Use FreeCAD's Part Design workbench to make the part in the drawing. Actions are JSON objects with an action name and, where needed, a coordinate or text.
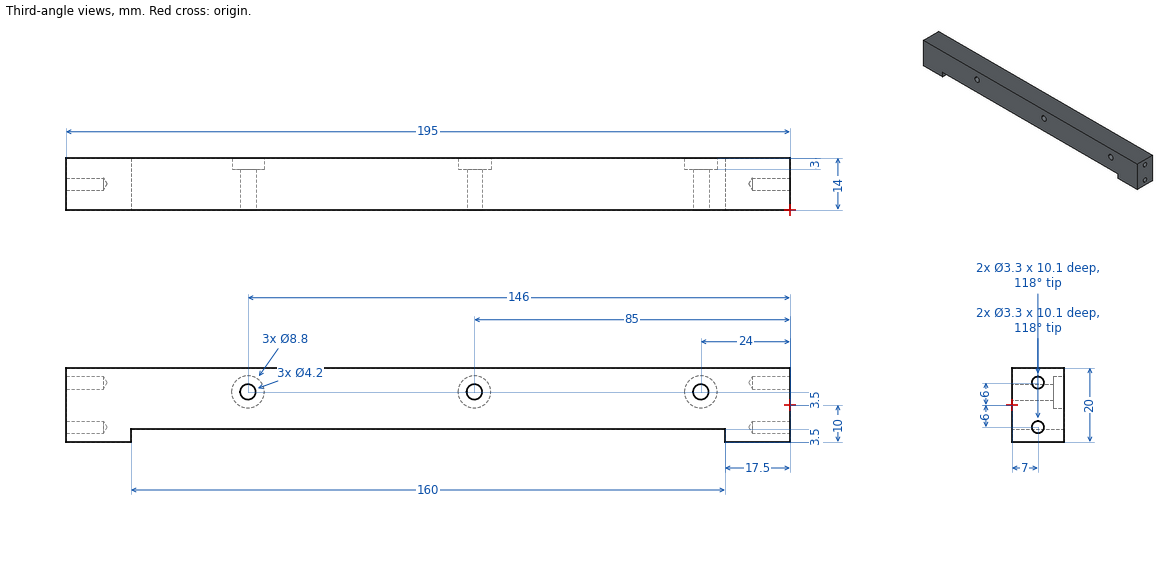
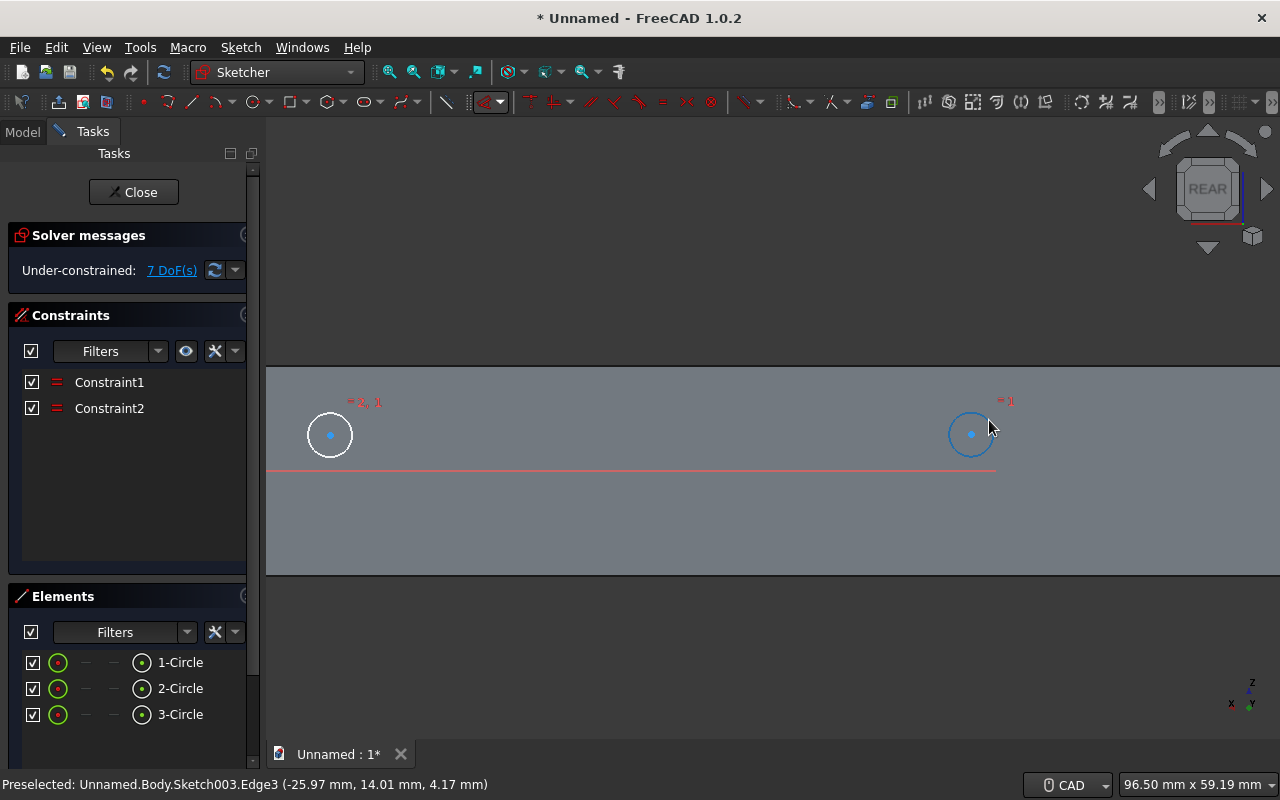
{"action": "left_click", "coordinate": [987, 419]}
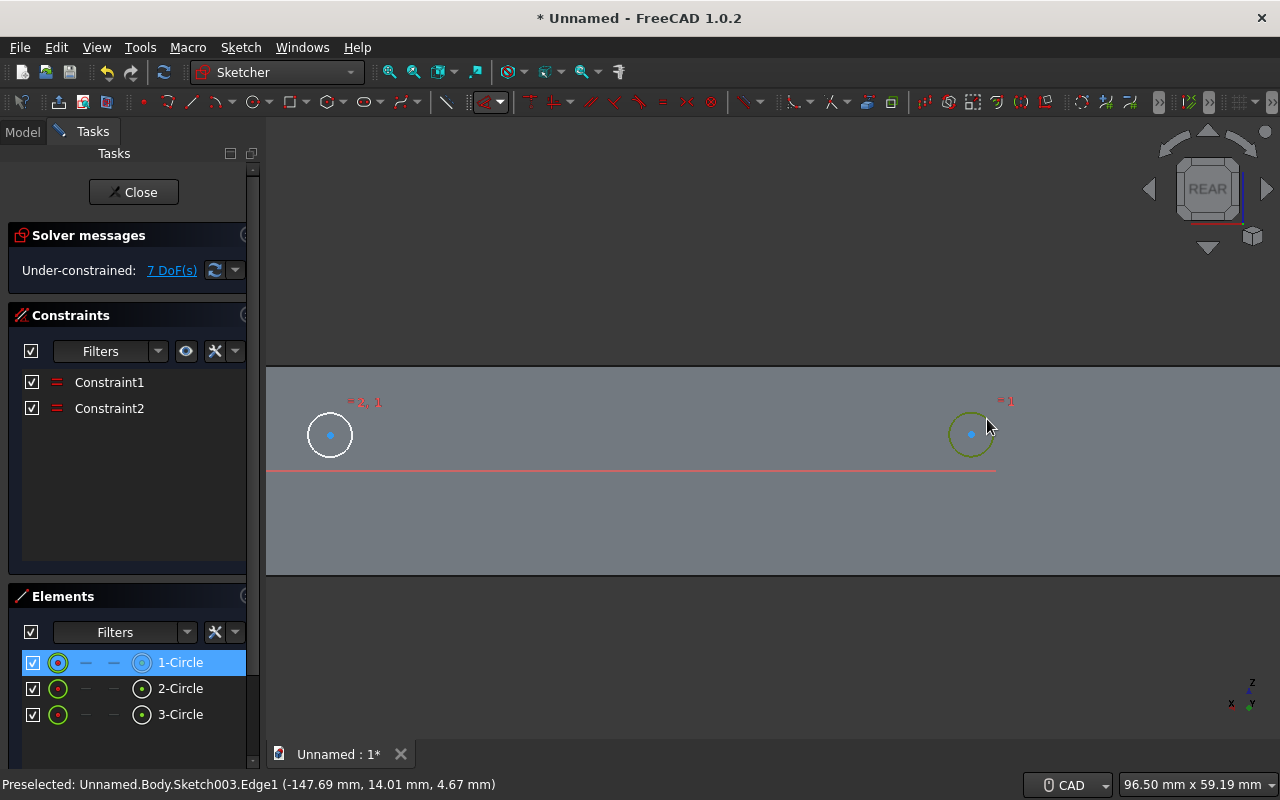
{"action": "key", "text": "k o"}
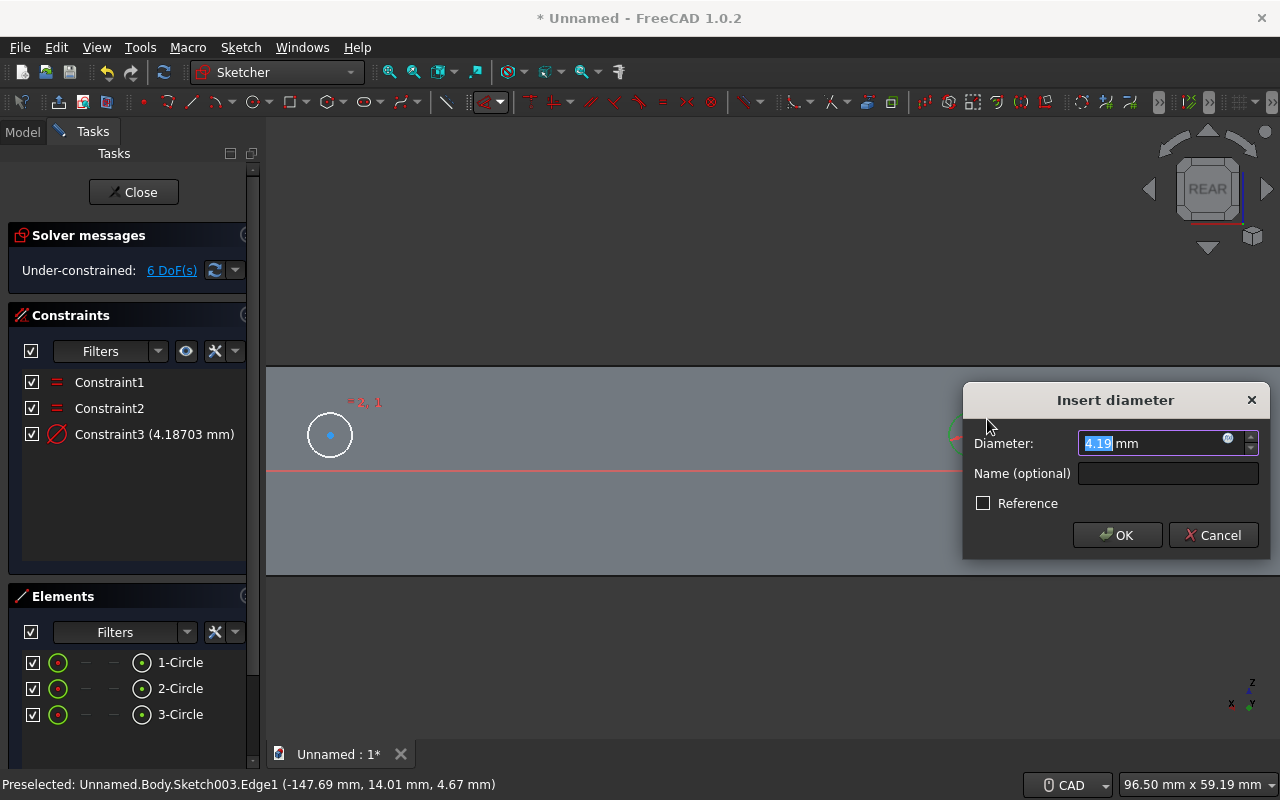
{"action": "type", "text": "4.2"}
{"action": "key", "text": "Return"}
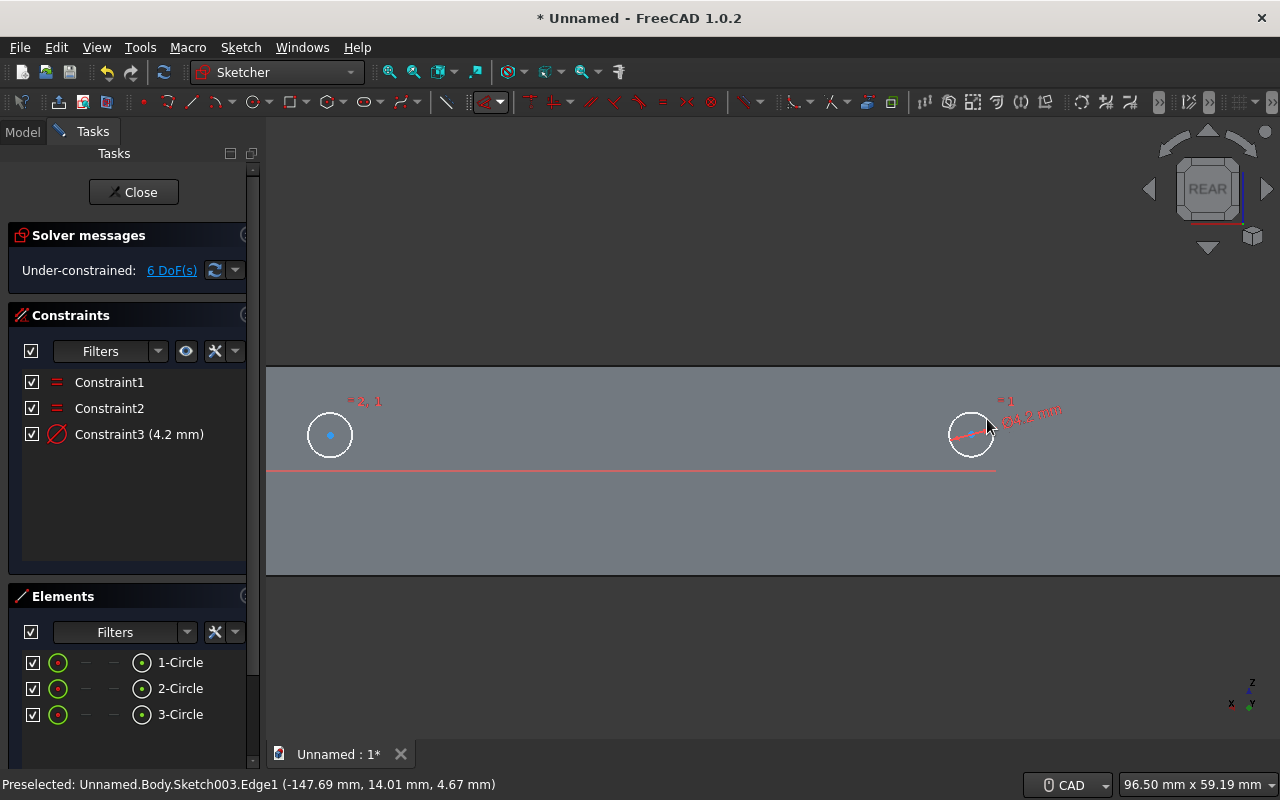
{"action": "left_click", "coordinate": [330, 435]}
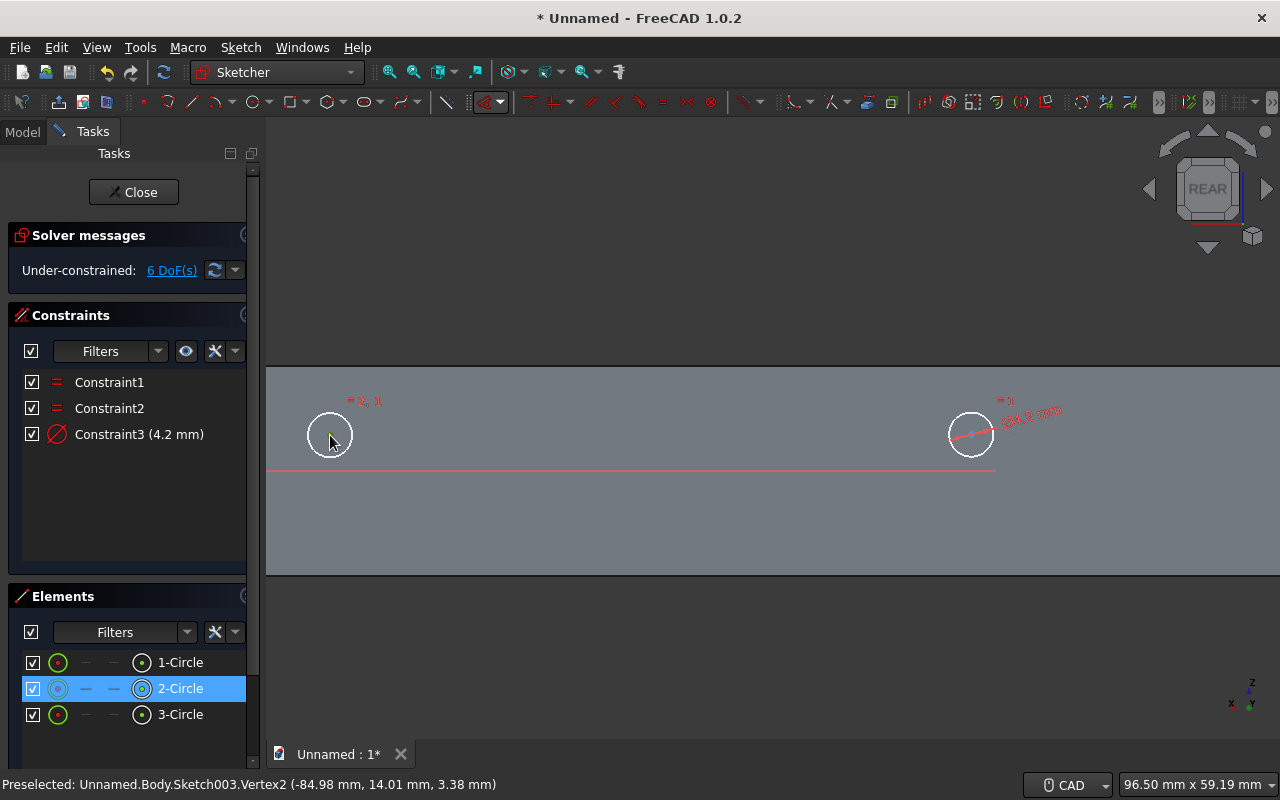
{"action": "key", "text": "l"}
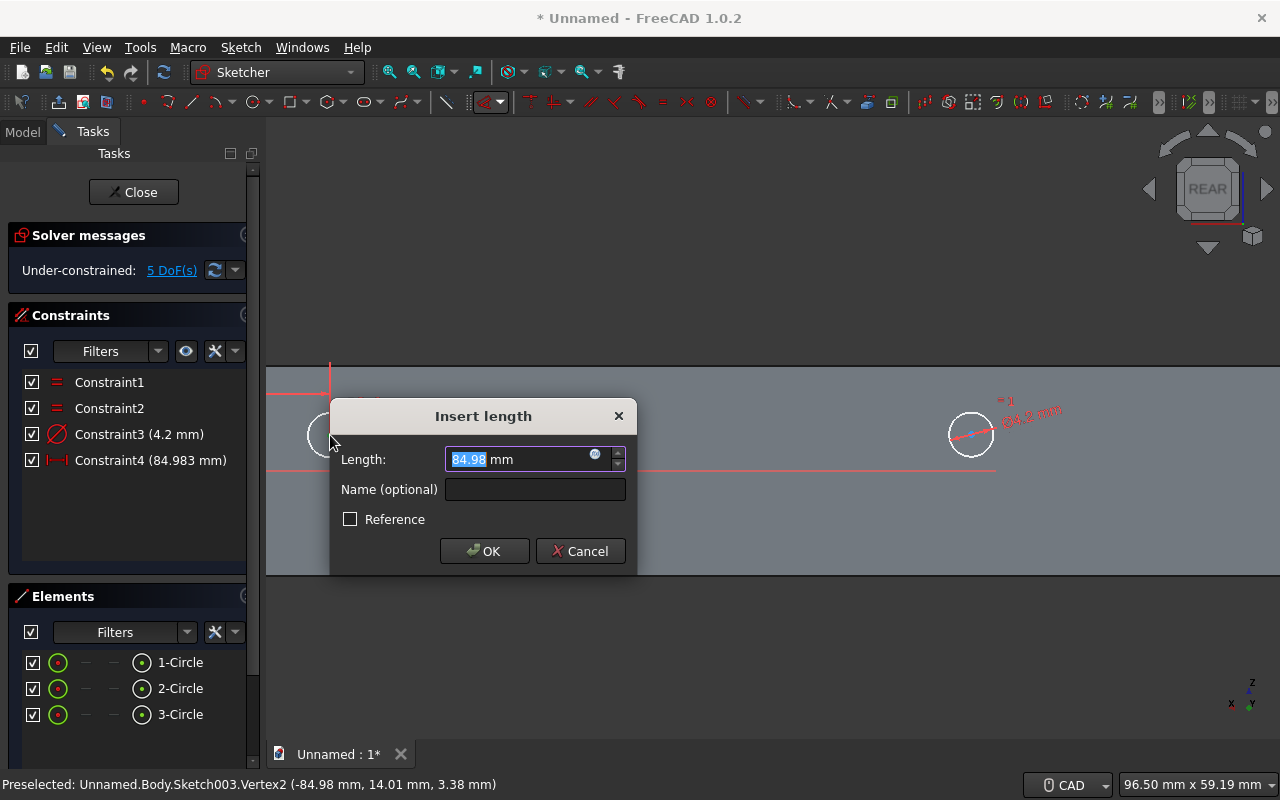
{"action": "type", "text": "85"}
{"action": "key", "text": "Return"}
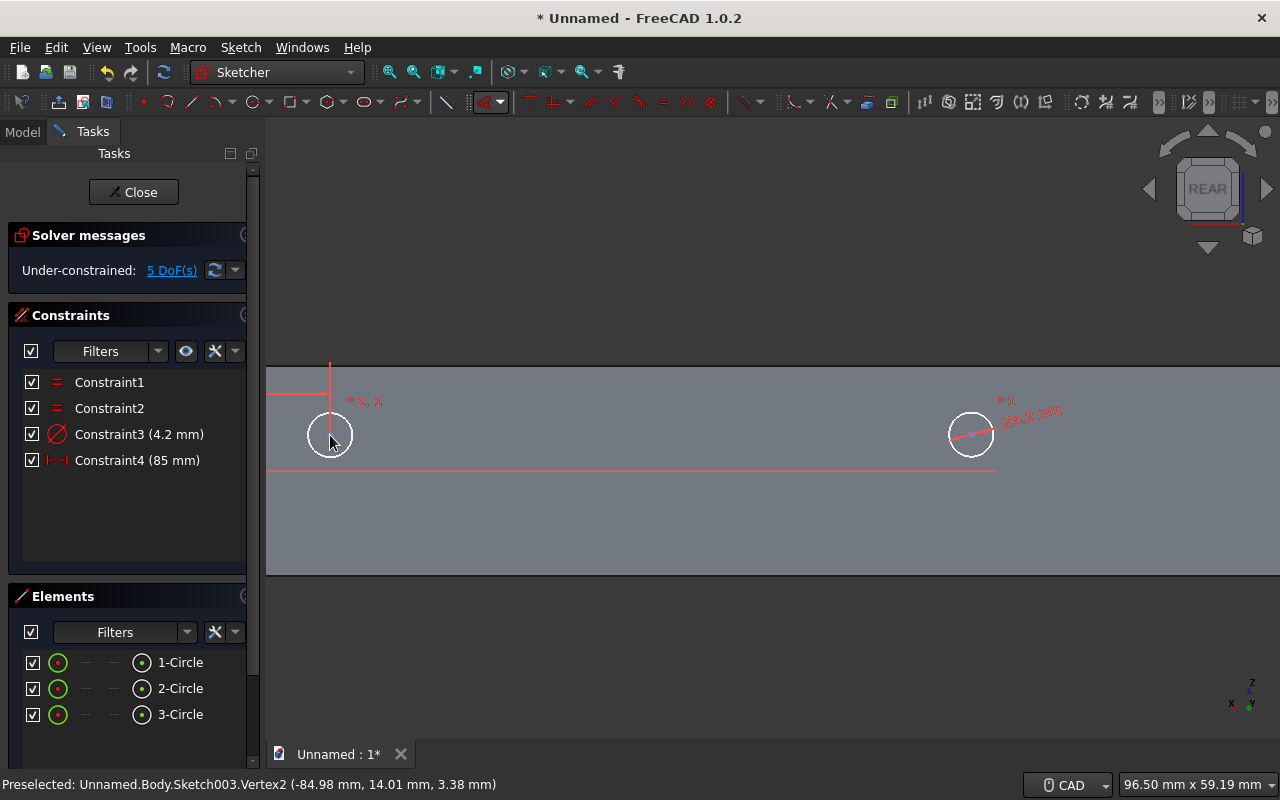
{"action": "scroll", "coordinate": [989, 420], "scroll_direction": "down", "scroll_amount": 5}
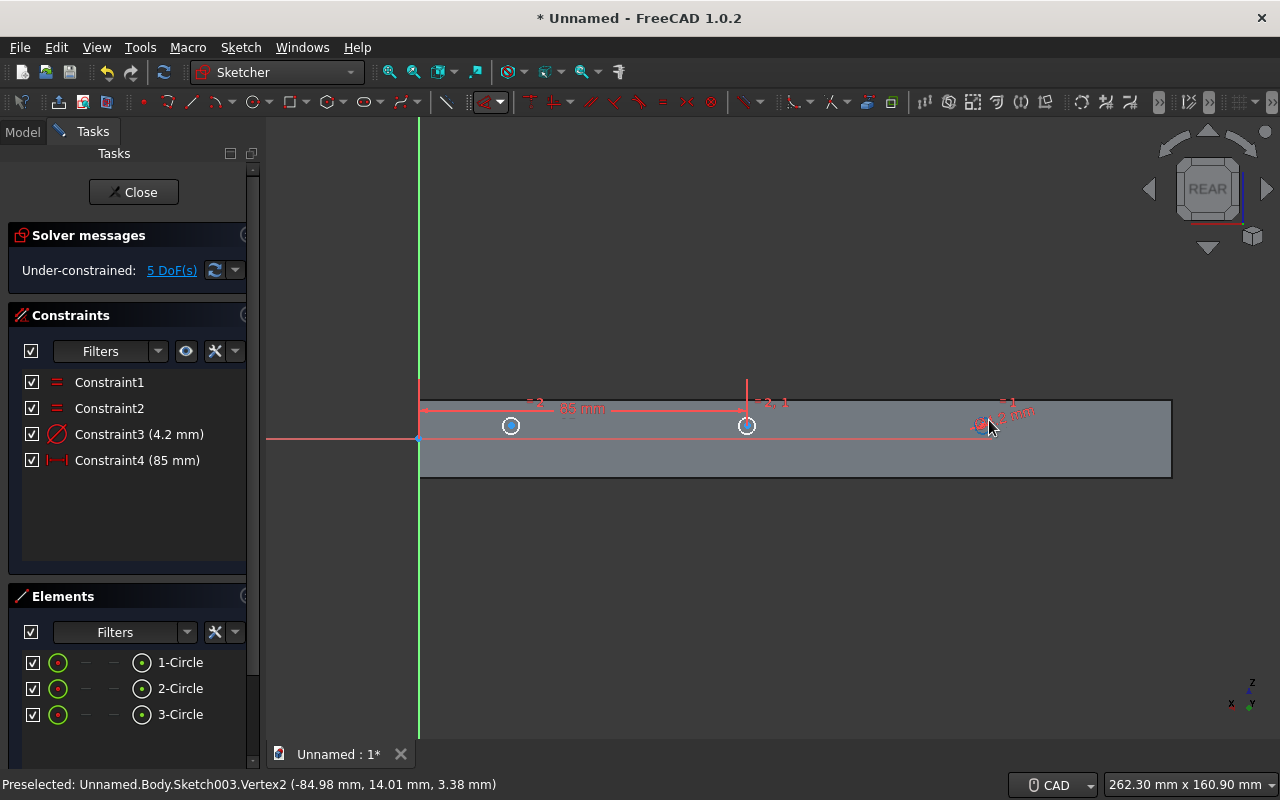
{"action": "left_click", "coordinate": [511, 426]}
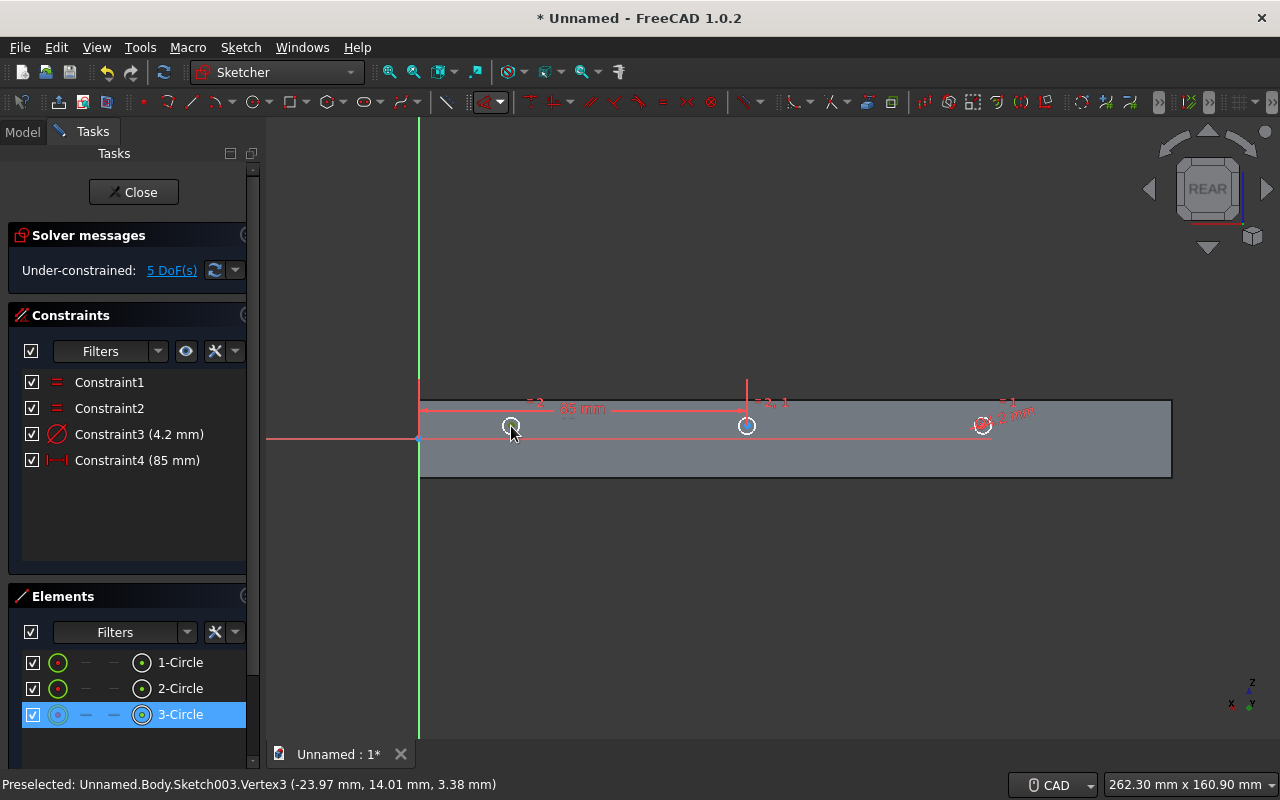
{"action": "key", "text": "l"}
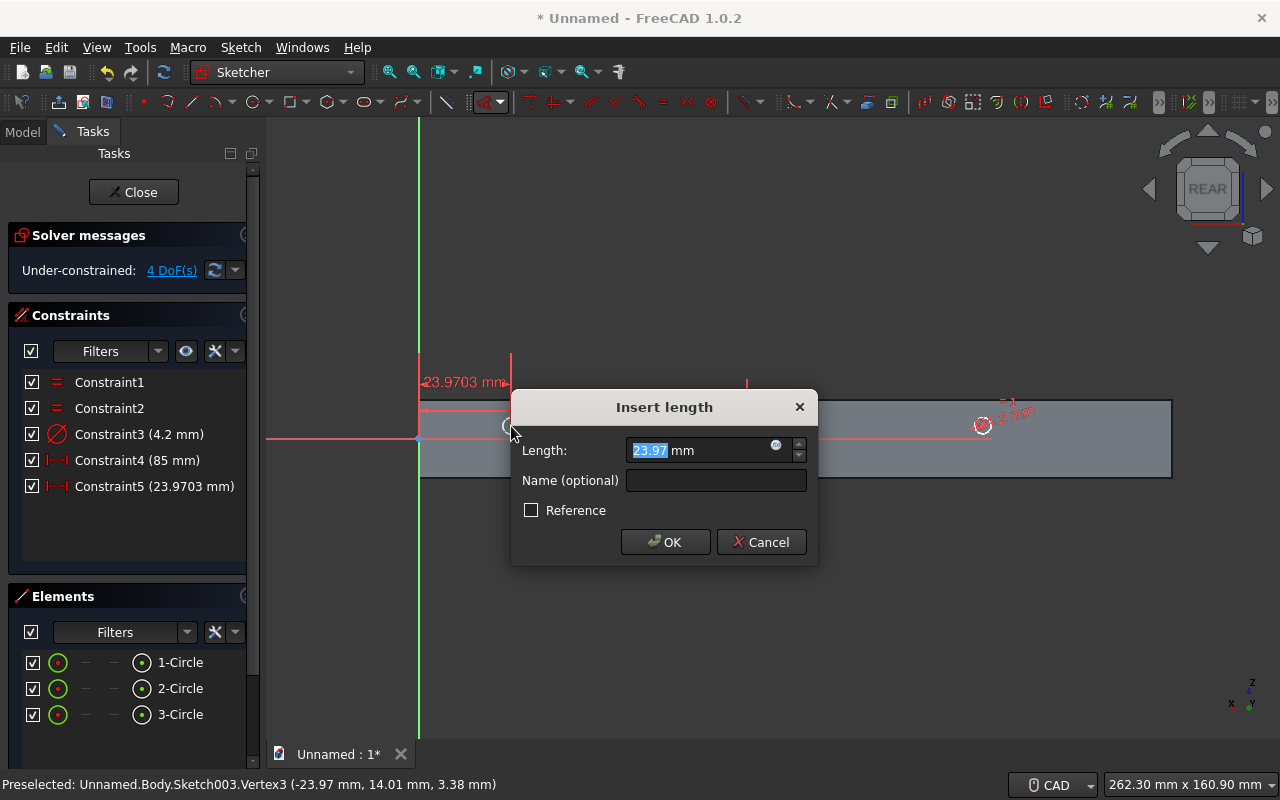
{"action": "type", "text": "24"}
{"action": "key", "text": "Return"}